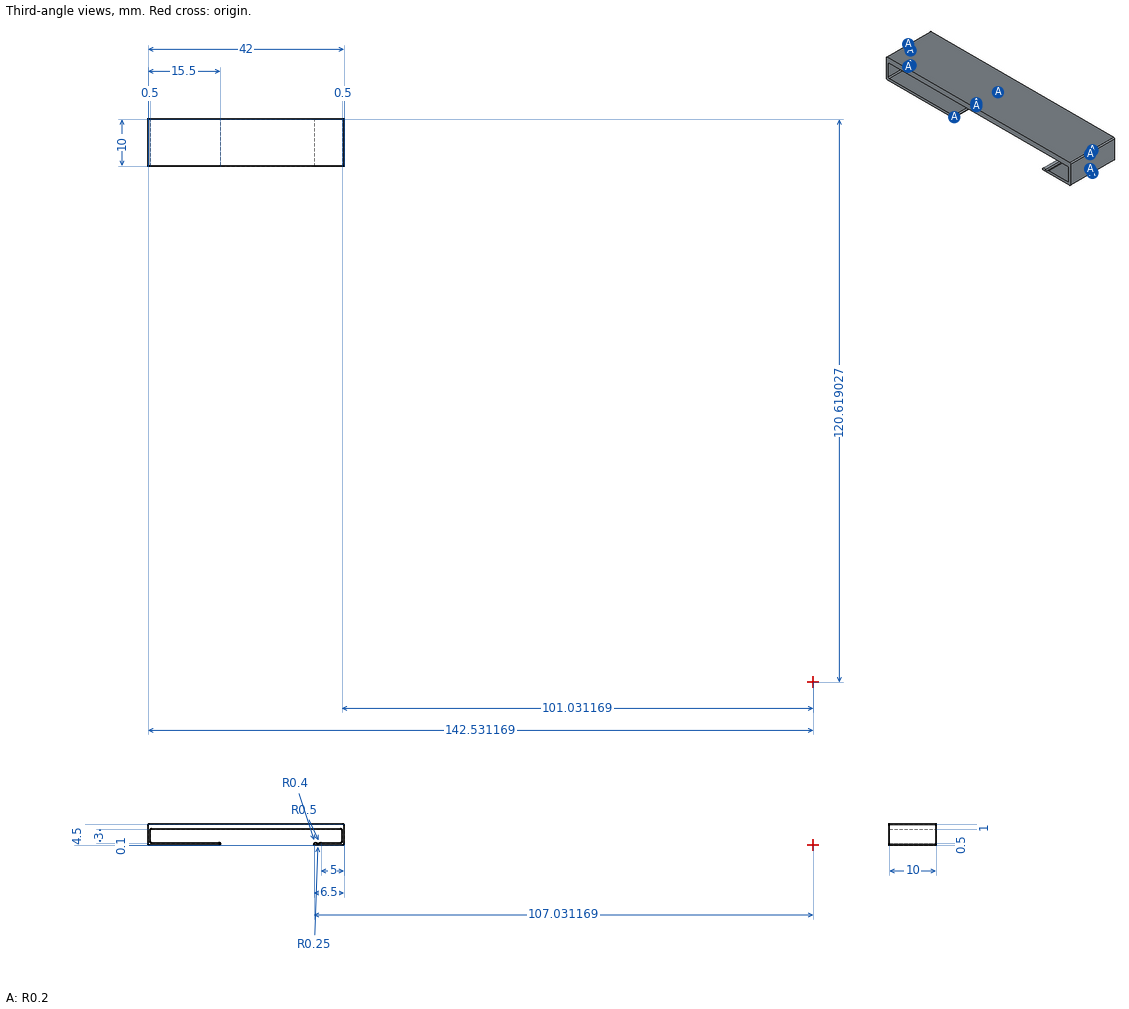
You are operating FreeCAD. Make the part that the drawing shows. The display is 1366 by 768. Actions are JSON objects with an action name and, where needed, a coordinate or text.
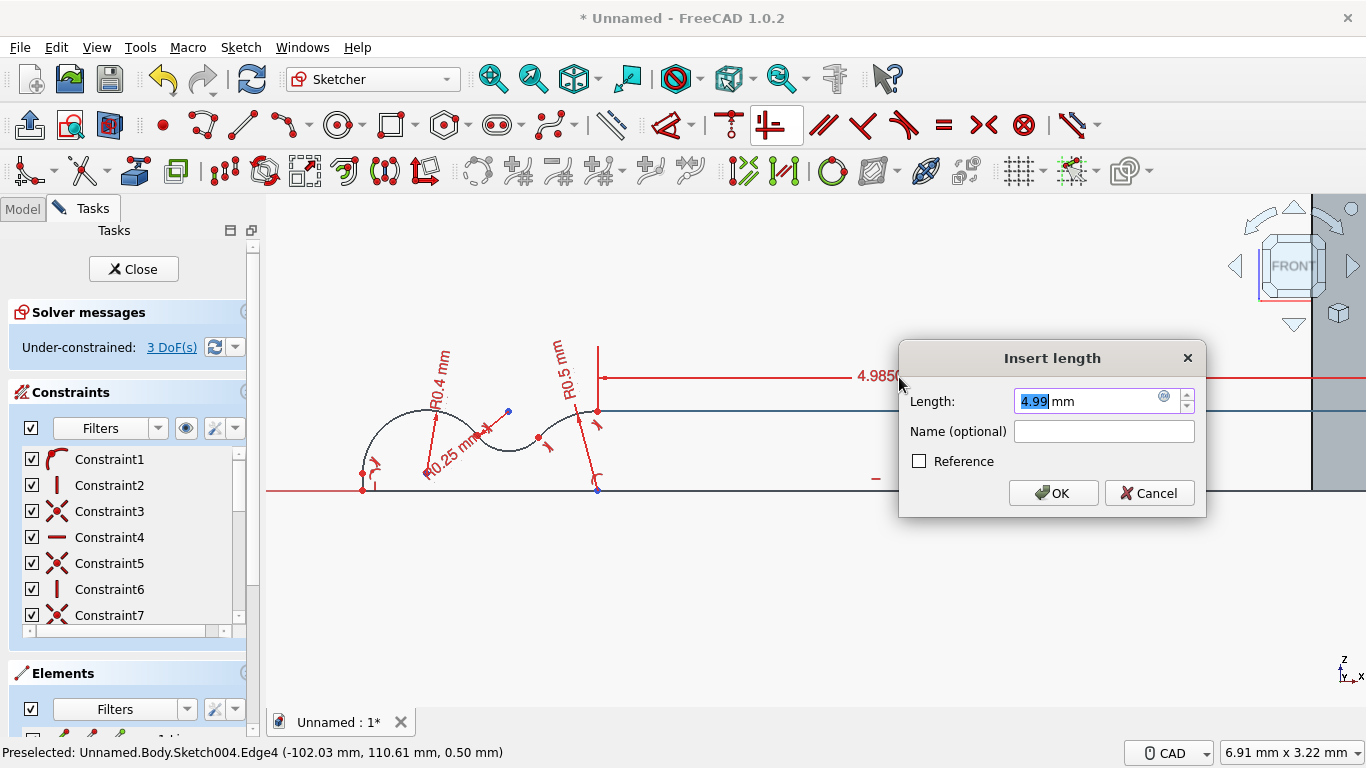
{"action": "type", "text": "5"}
{"action": "key", "text": "Return"}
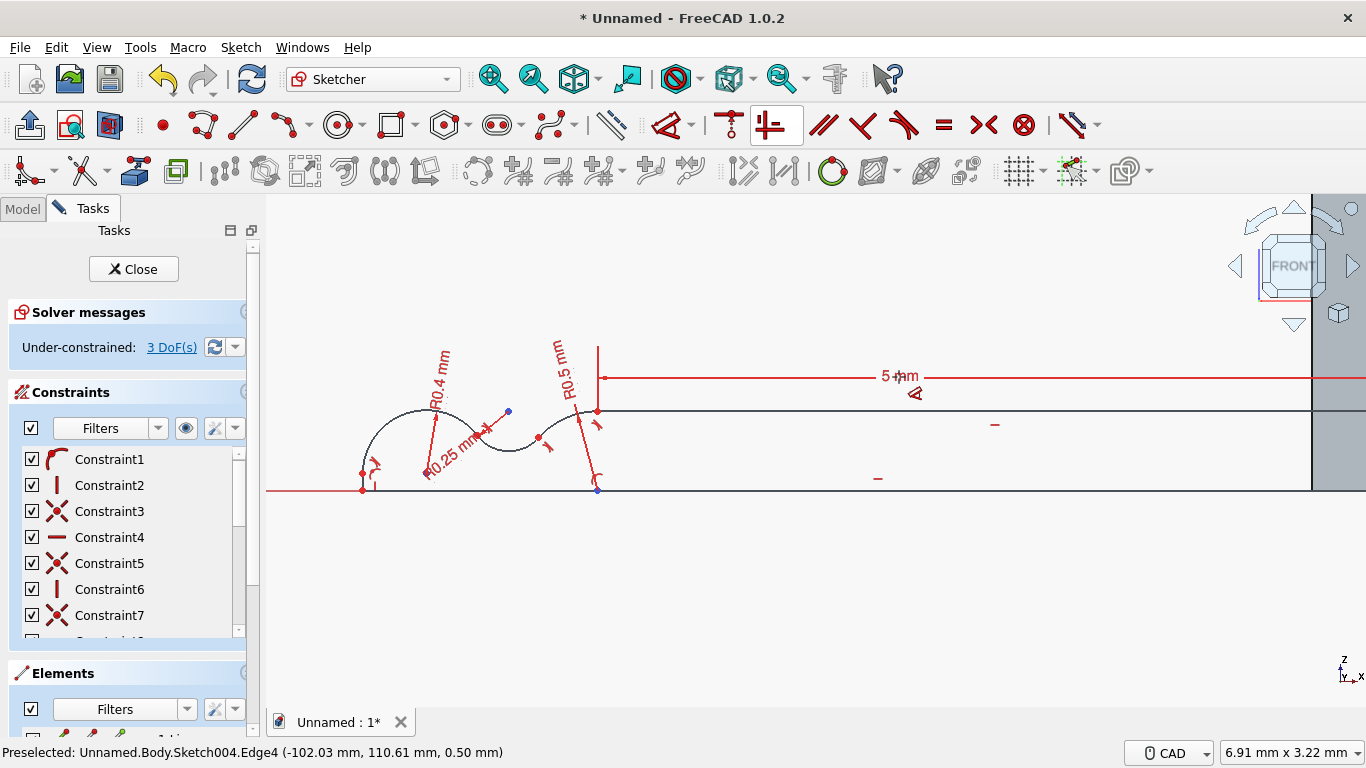
{"action": "scroll", "coordinate": [363, 482], "scroll_direction": "up", "scroll_amount": 5}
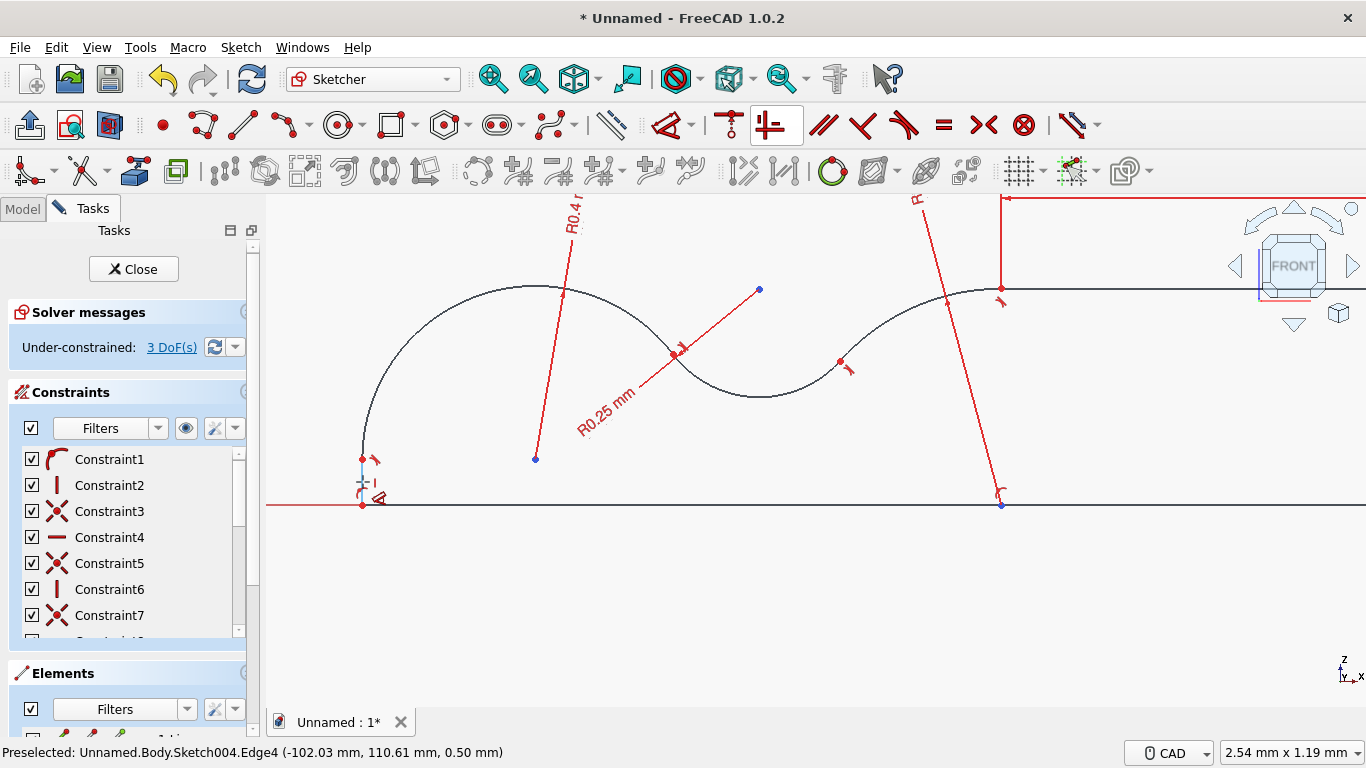
{"action": "left_click", "coordinate": [362, 482]}
{"action": "left_click", "coordinate": [328, 482]}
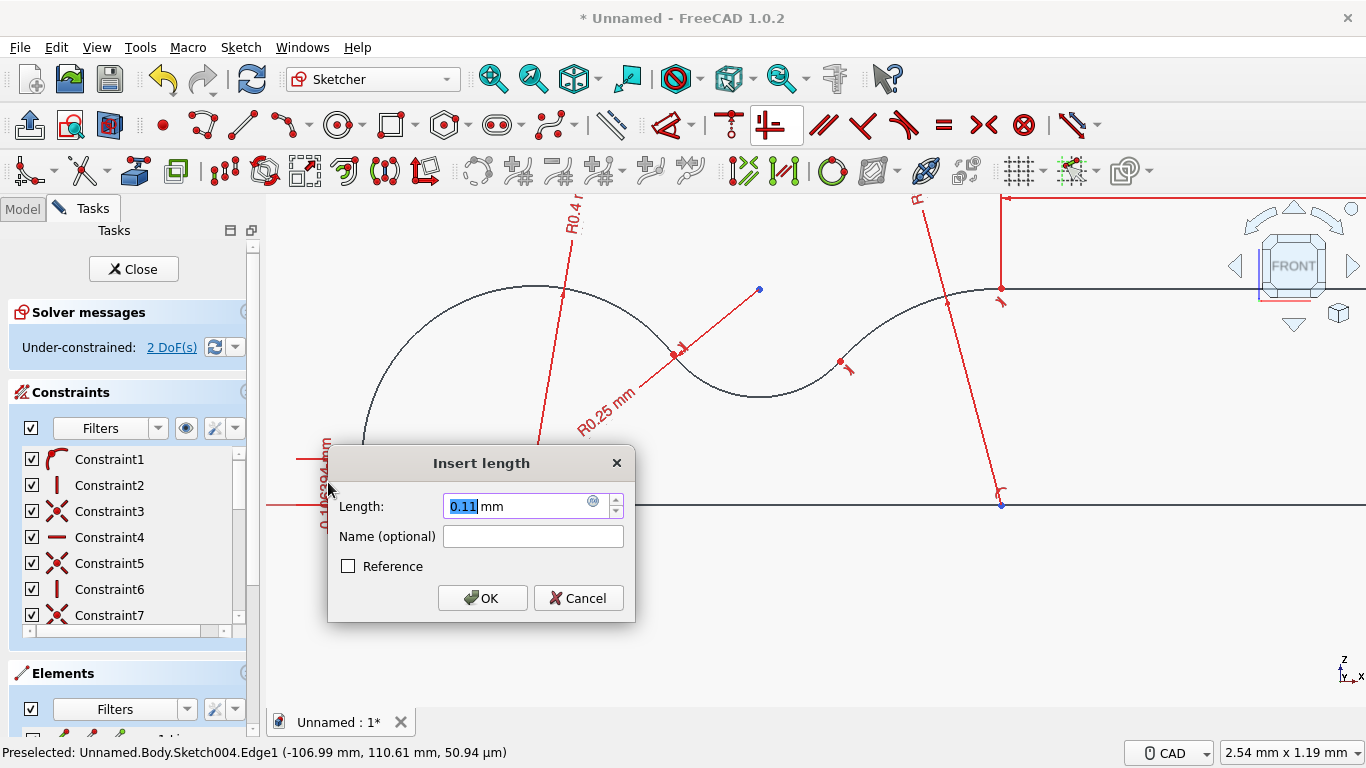
{"action": "type", "text": "0.1"}
{"action": "key", "text": "Return"}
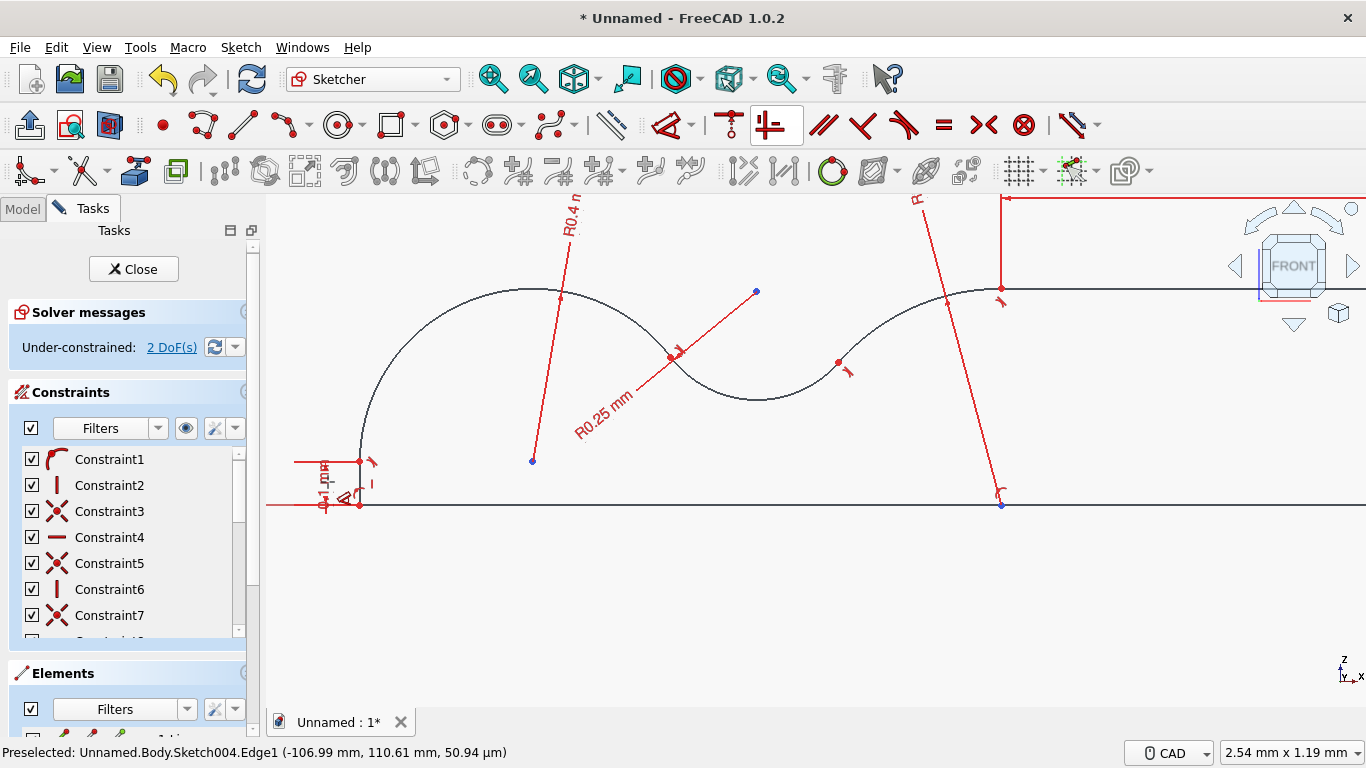
{"action": "scroll", "coordinate": [419, 468], "scroll_direction": "down", "scroll_amount": 7}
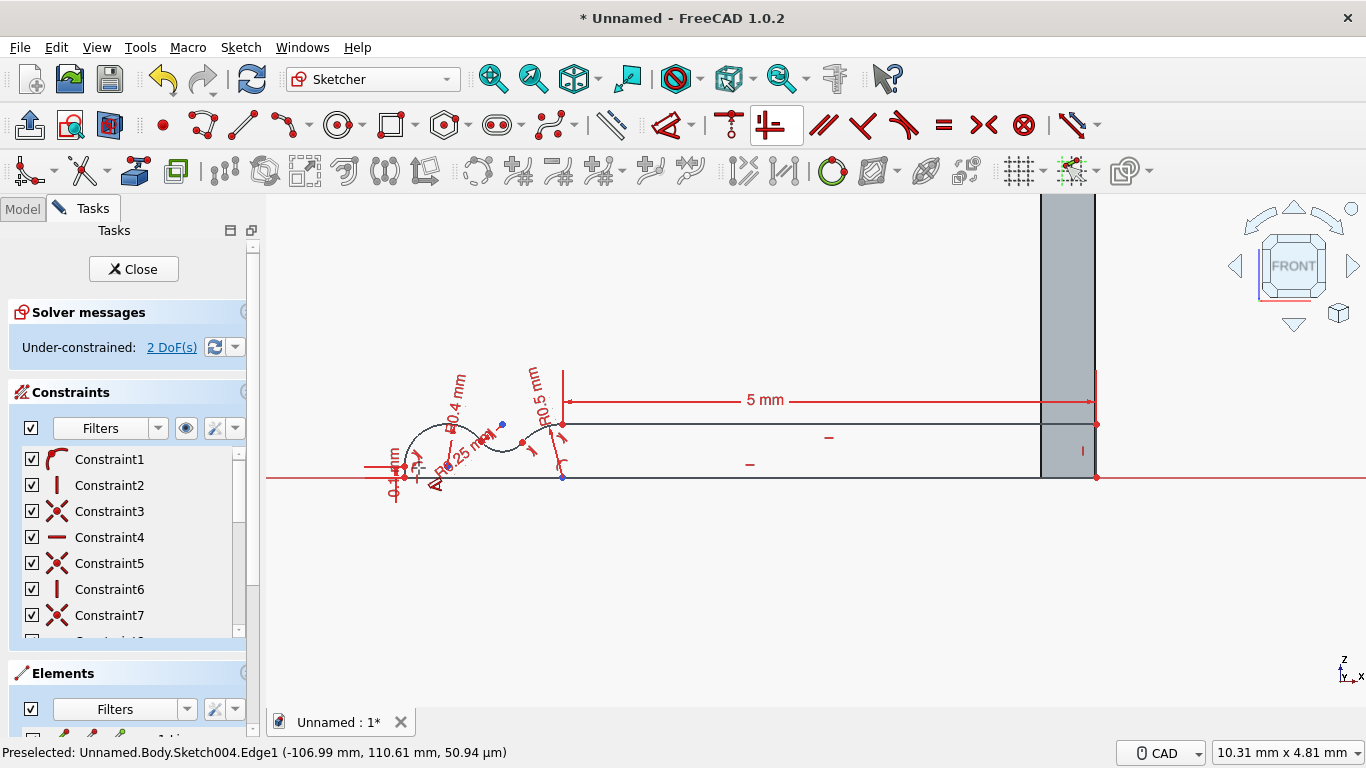
{"action": "left_click", "coordinate": [543, 478]}
{"action": "left_click", "coordinate": [750, 512]}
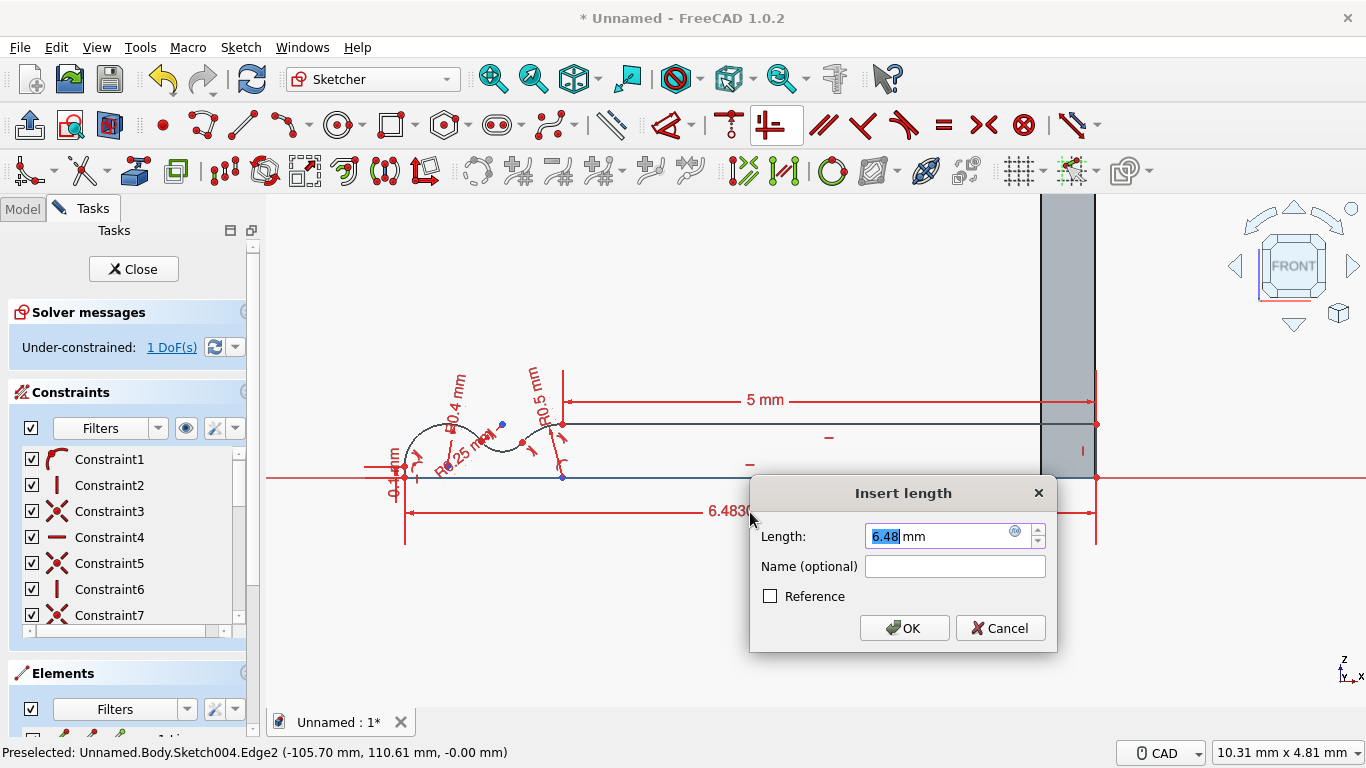
{"action": "type", "text": "6.5"}
{"action": "key", "text": "Return"}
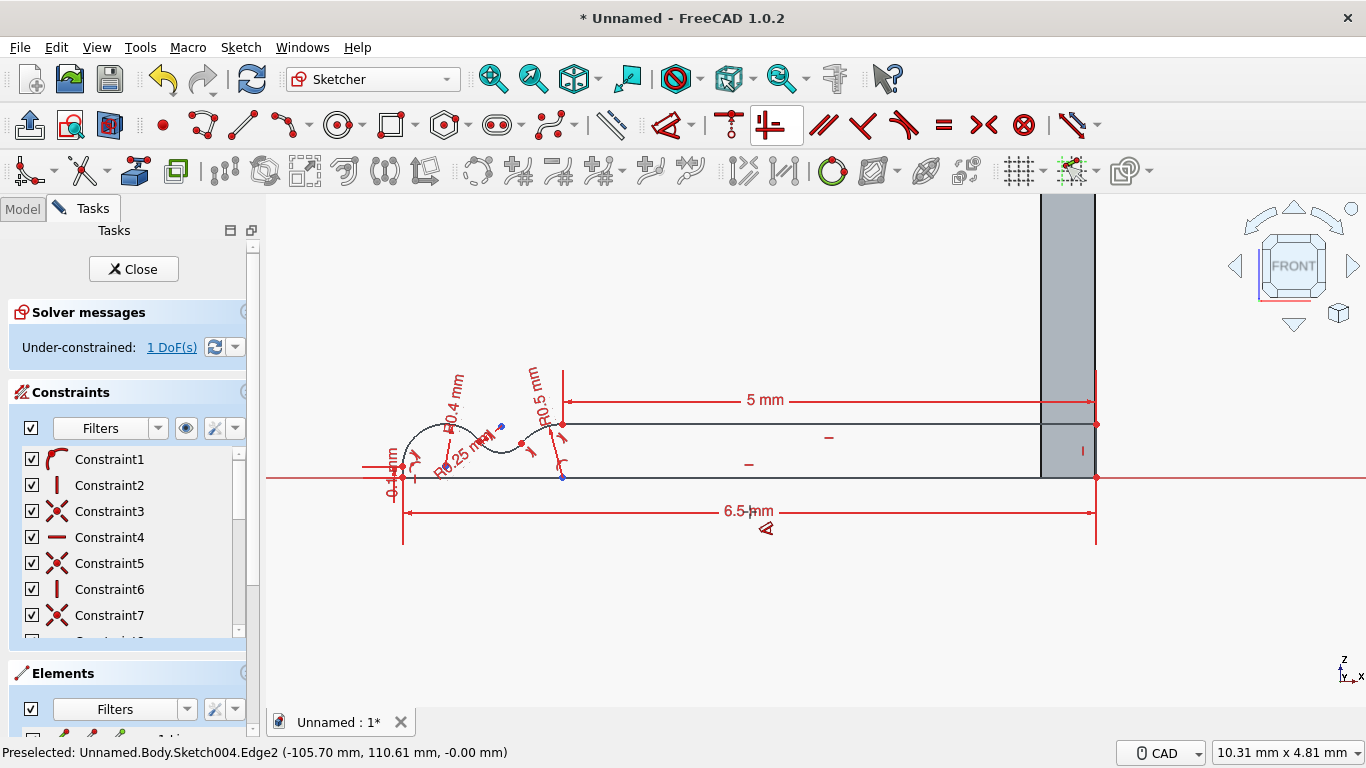
{"action": "left_click", "coordinate": [403, 467]}
{"action": "left_click", "coordinate": [618, 512]}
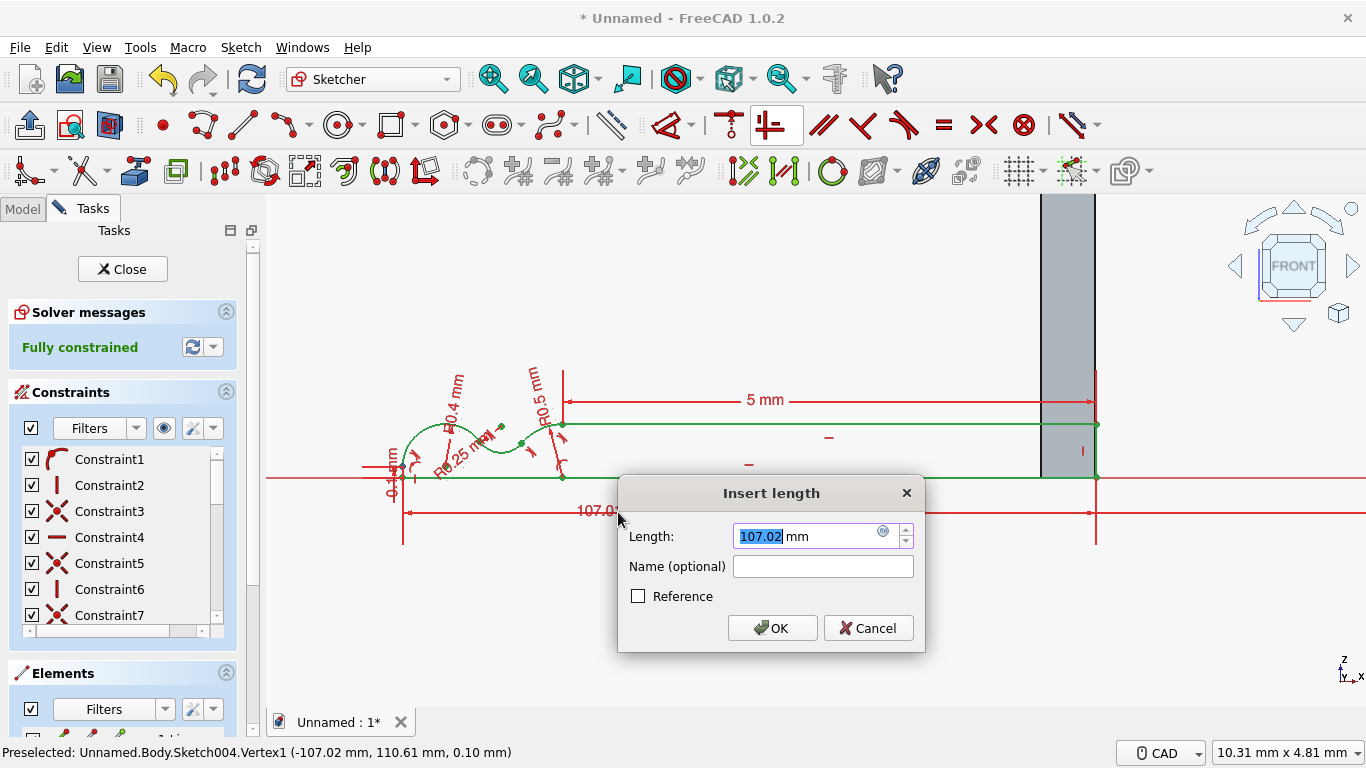
{"action": "type", "text": "107.031169"}
{"action": "key", "text": "Return"}
{"action": "key", "text": "Escape"}